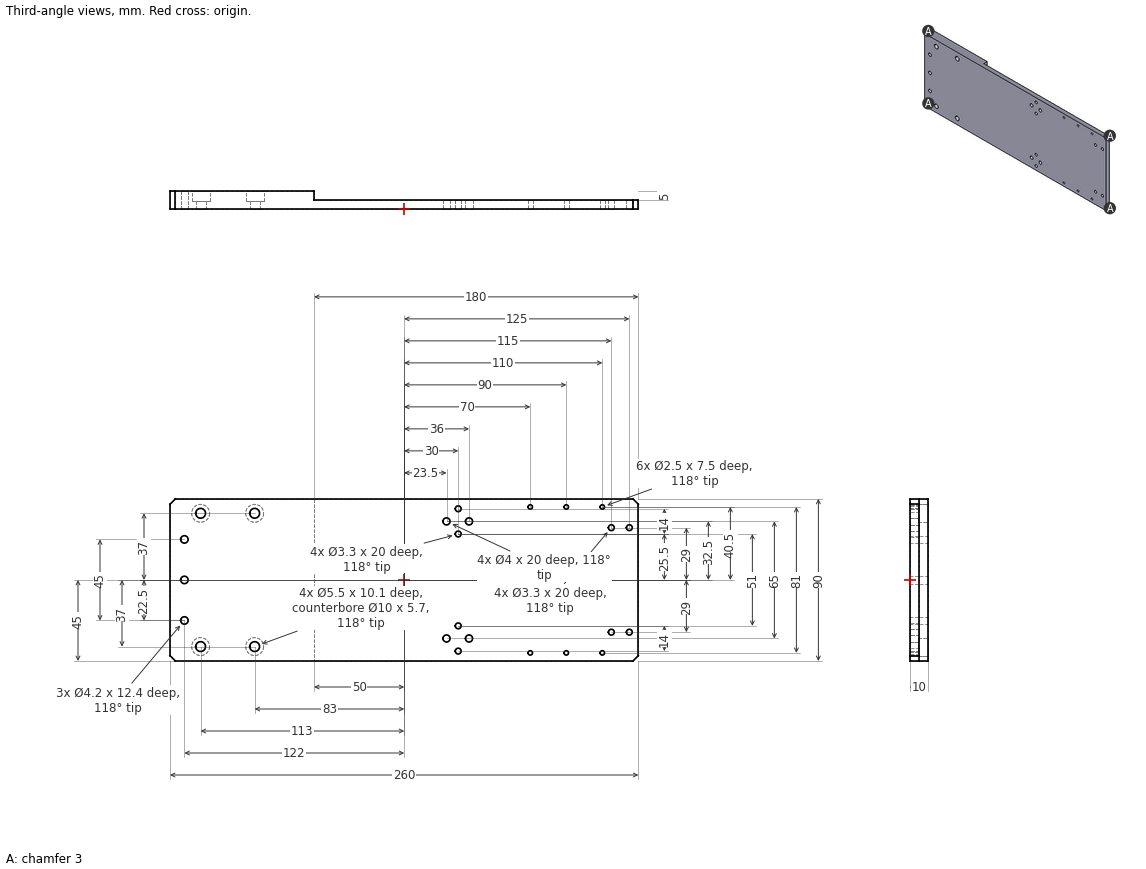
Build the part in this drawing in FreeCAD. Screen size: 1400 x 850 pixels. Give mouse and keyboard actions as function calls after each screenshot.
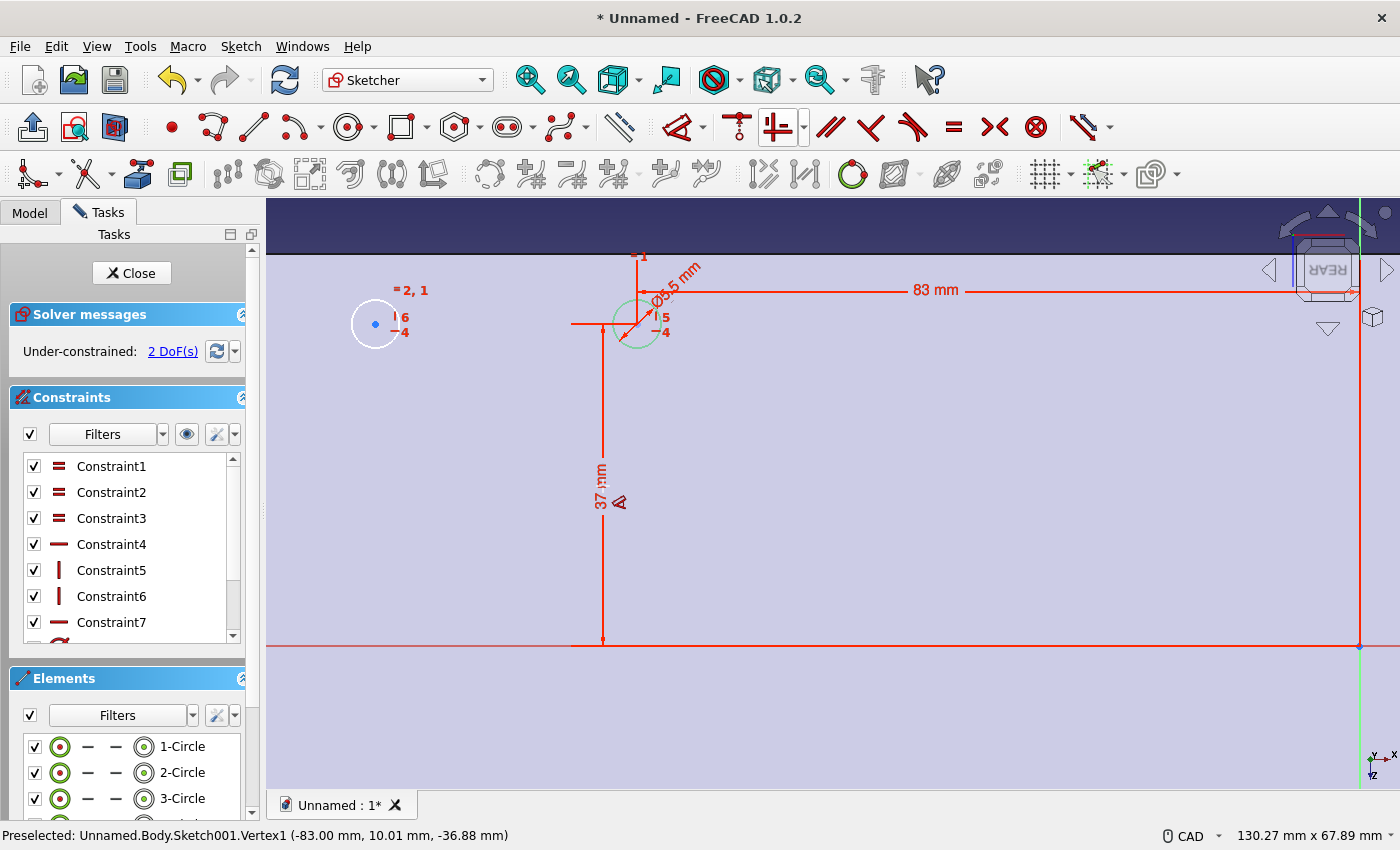
scroll(654, 308, down, 3)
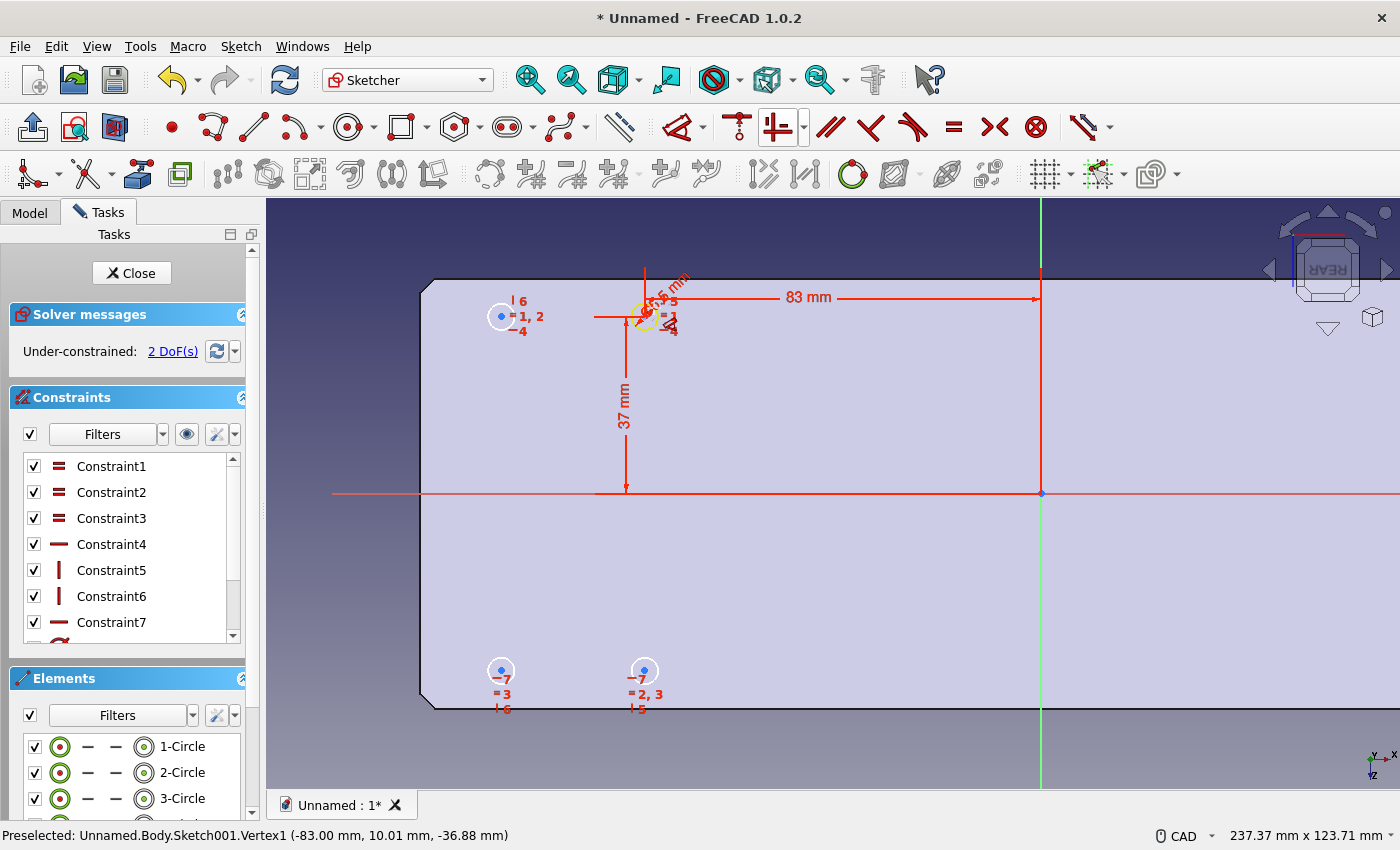
click(645, 671)
click(1075, 582)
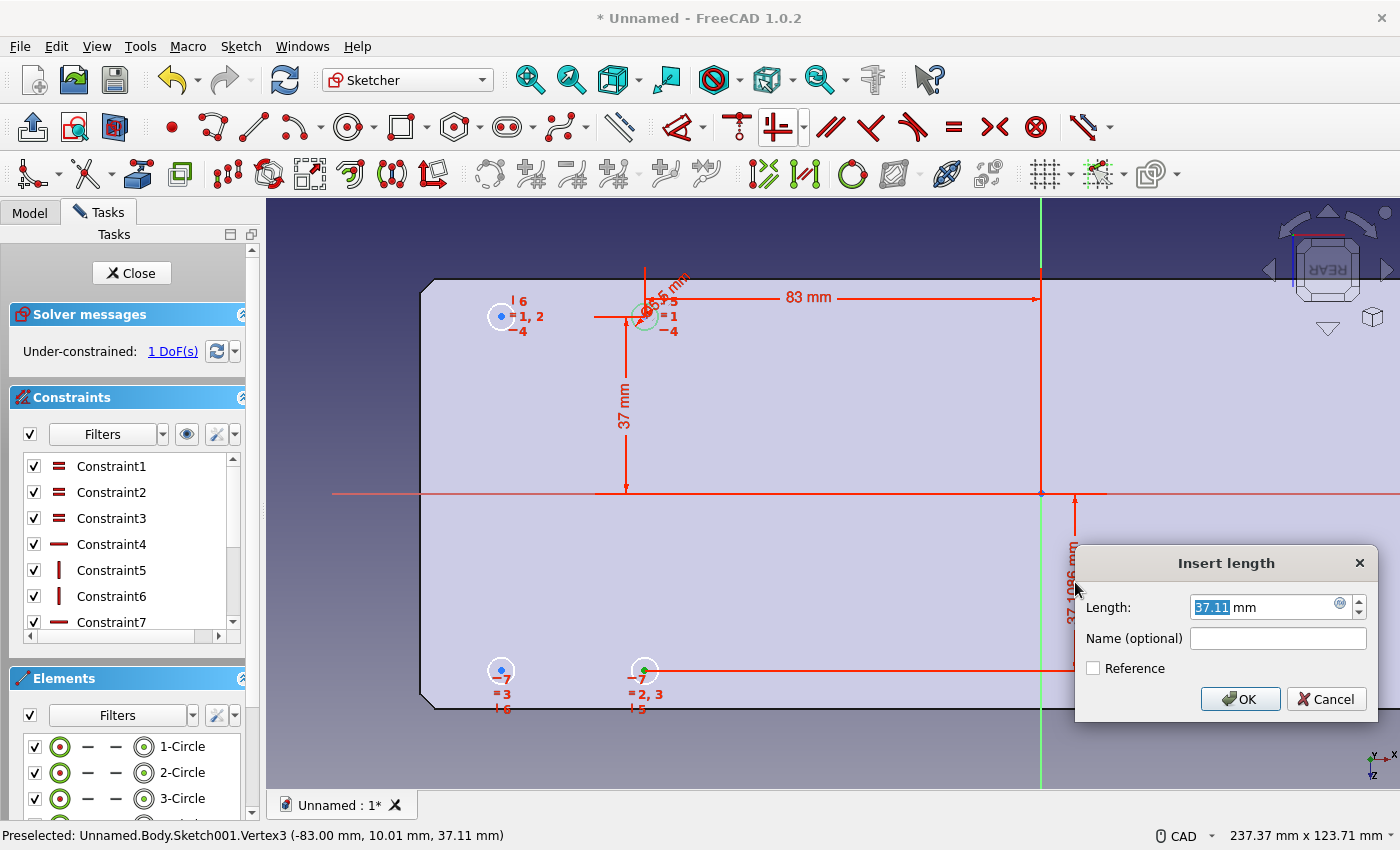
text(37)
key(Return)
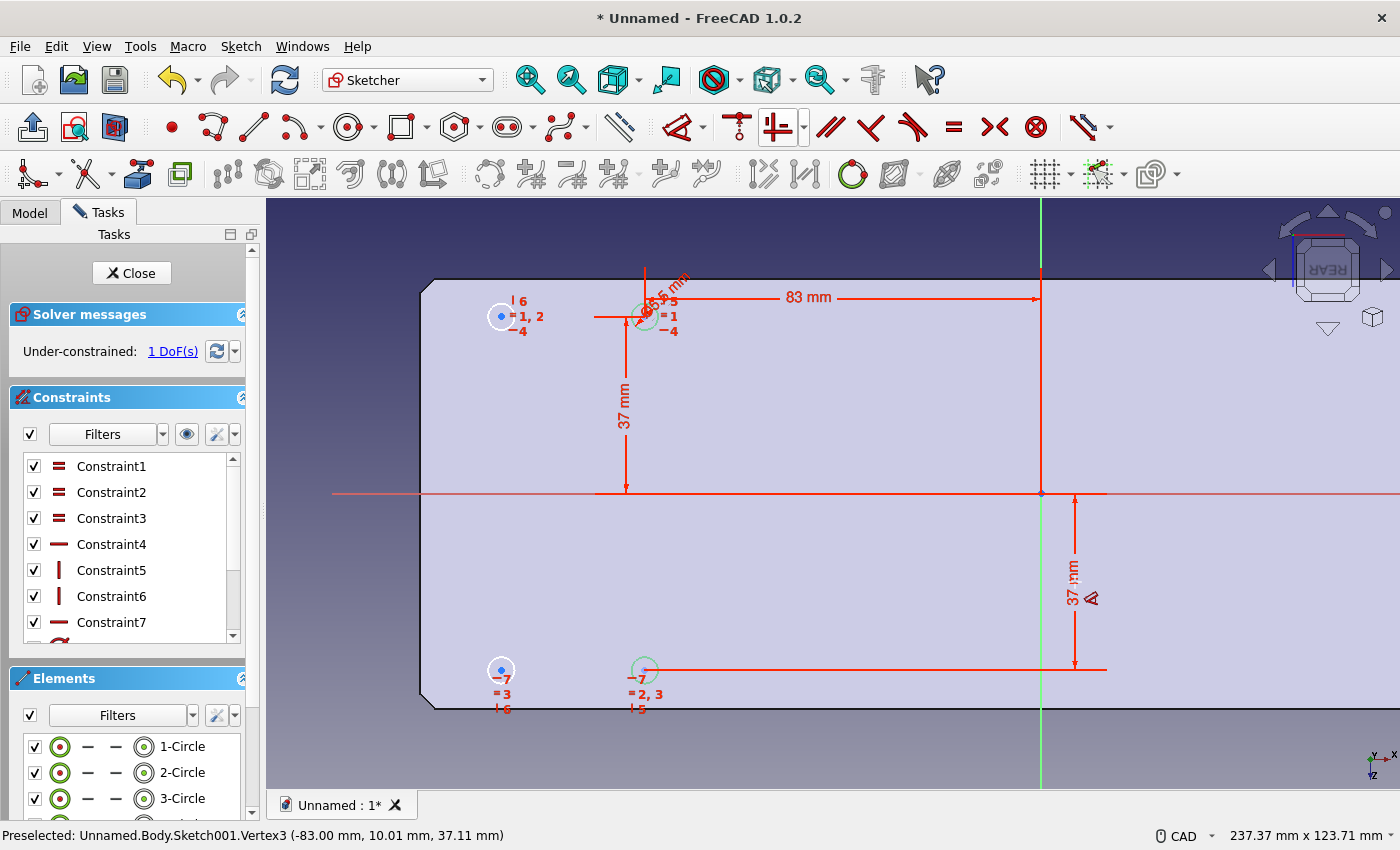
click(501, 317)
click(896, 283)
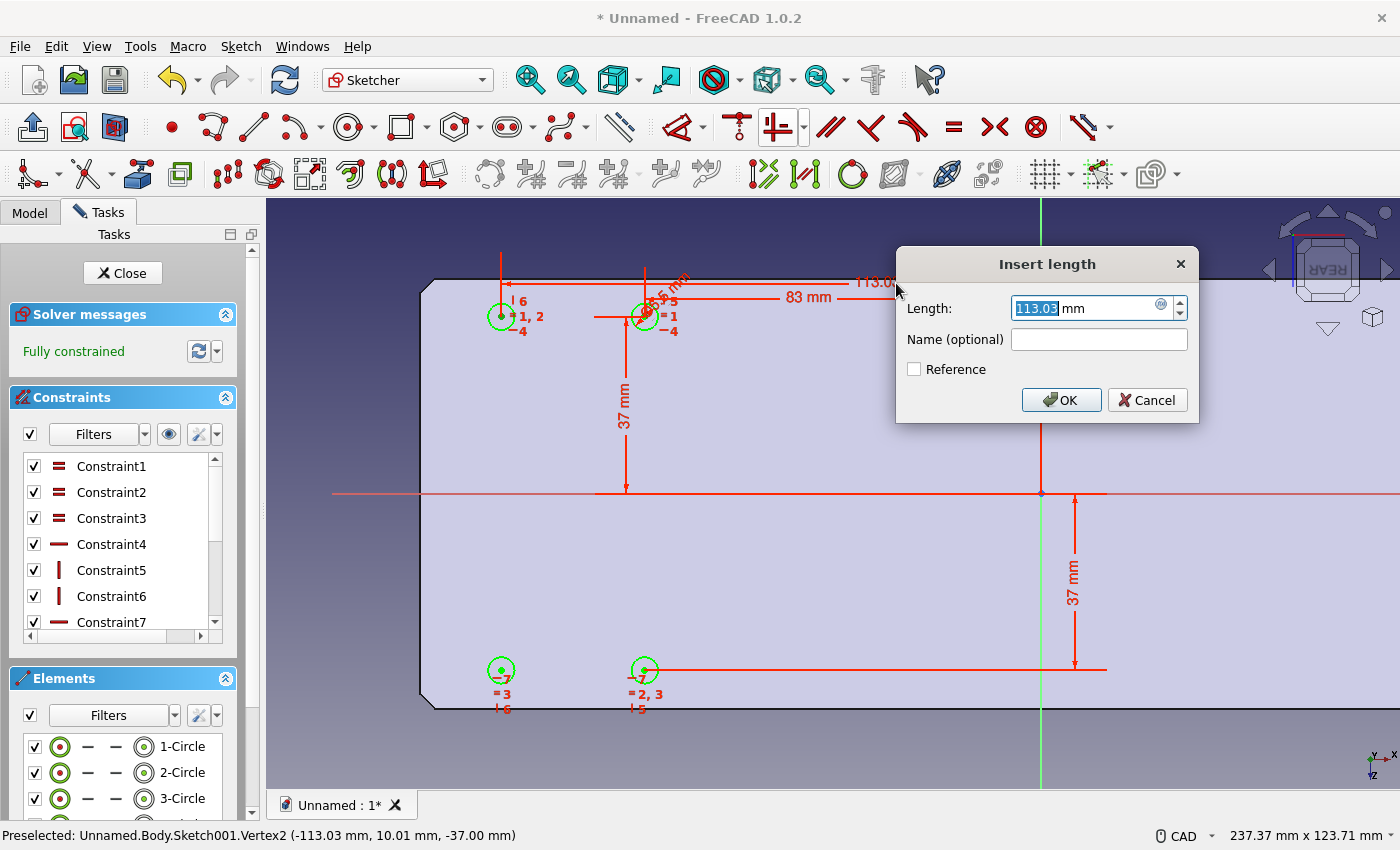
text(113)
key(Return)
key(Escape)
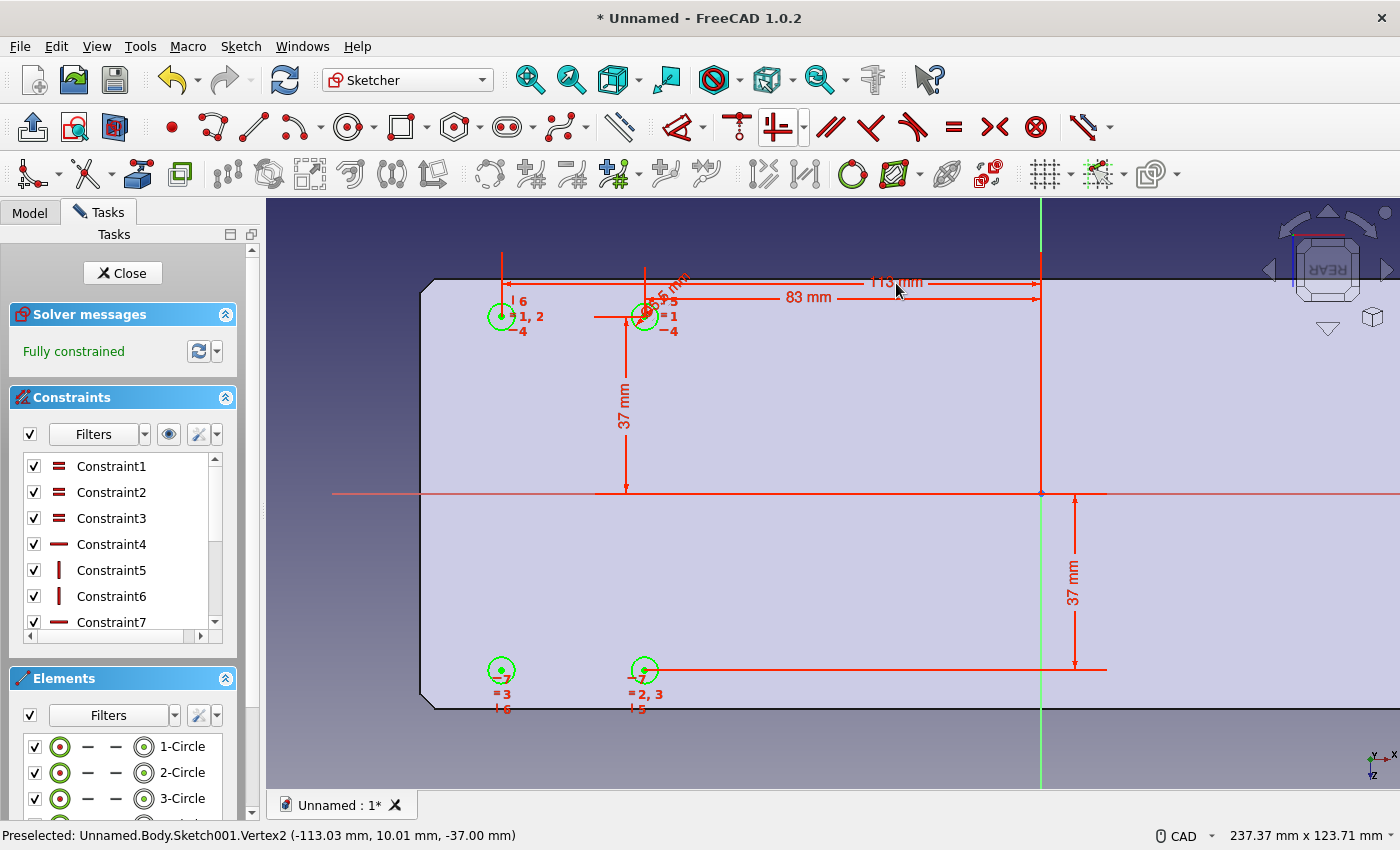
click(123, 273)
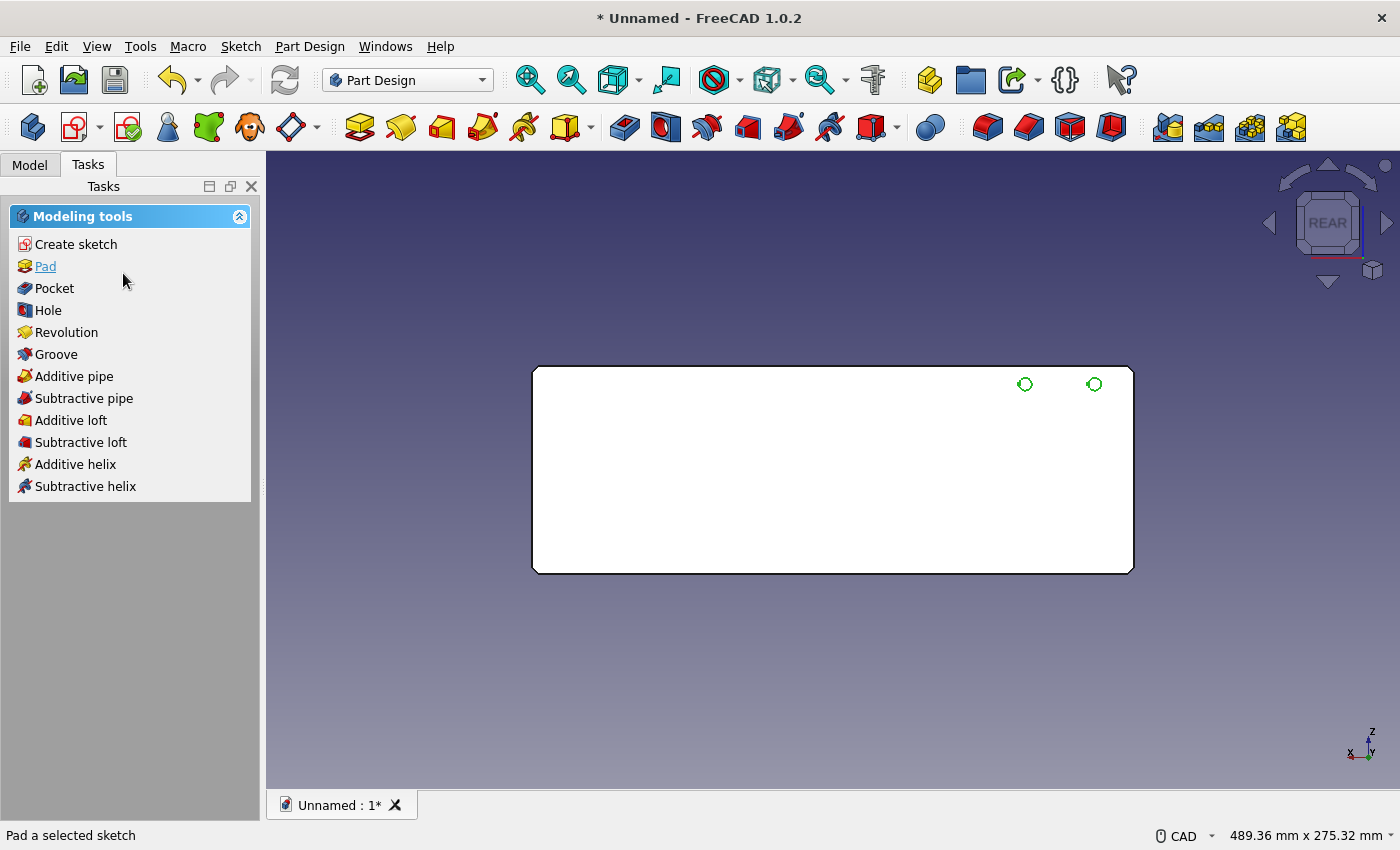
click(666, 128)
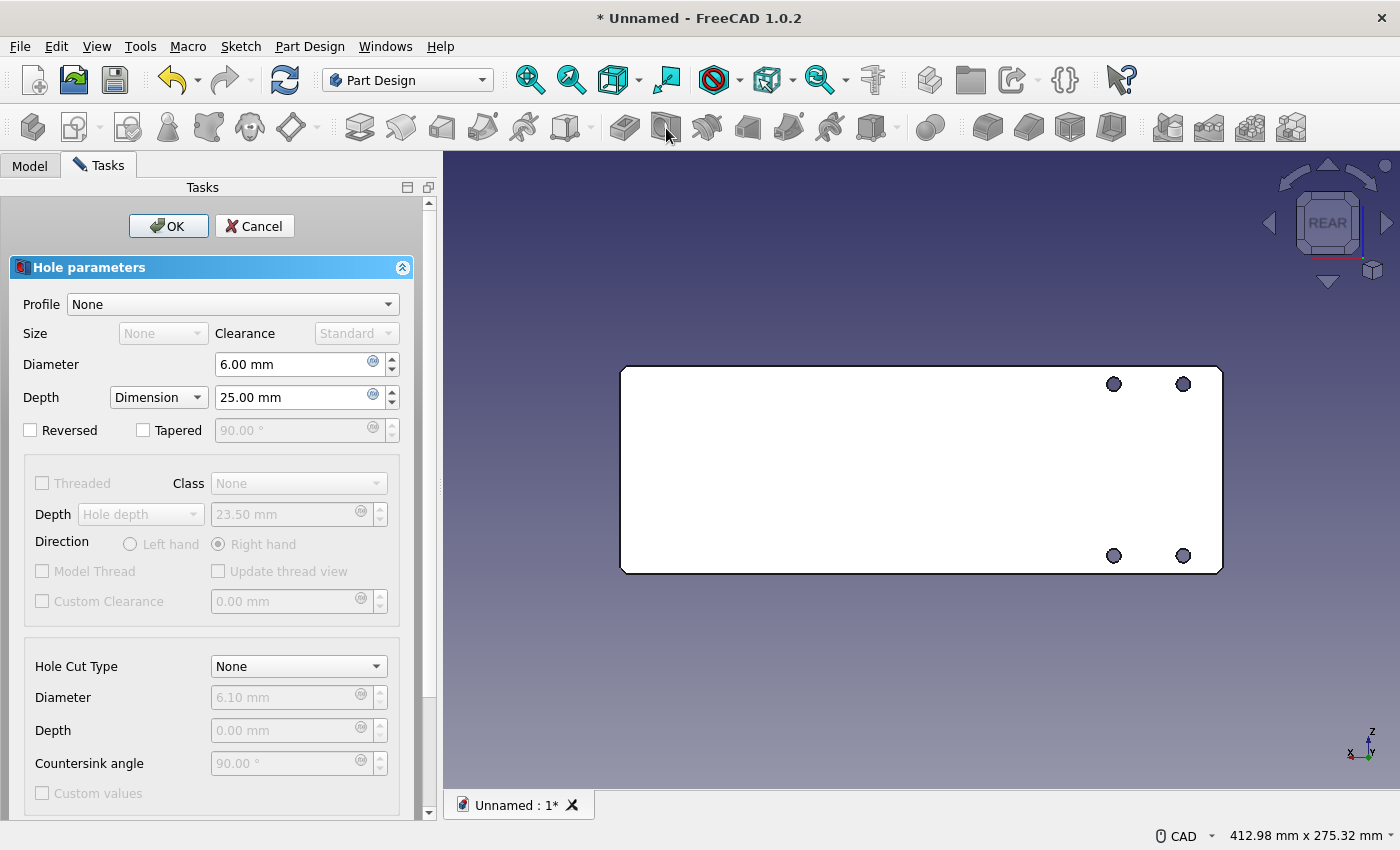
triple_click(300, 364)